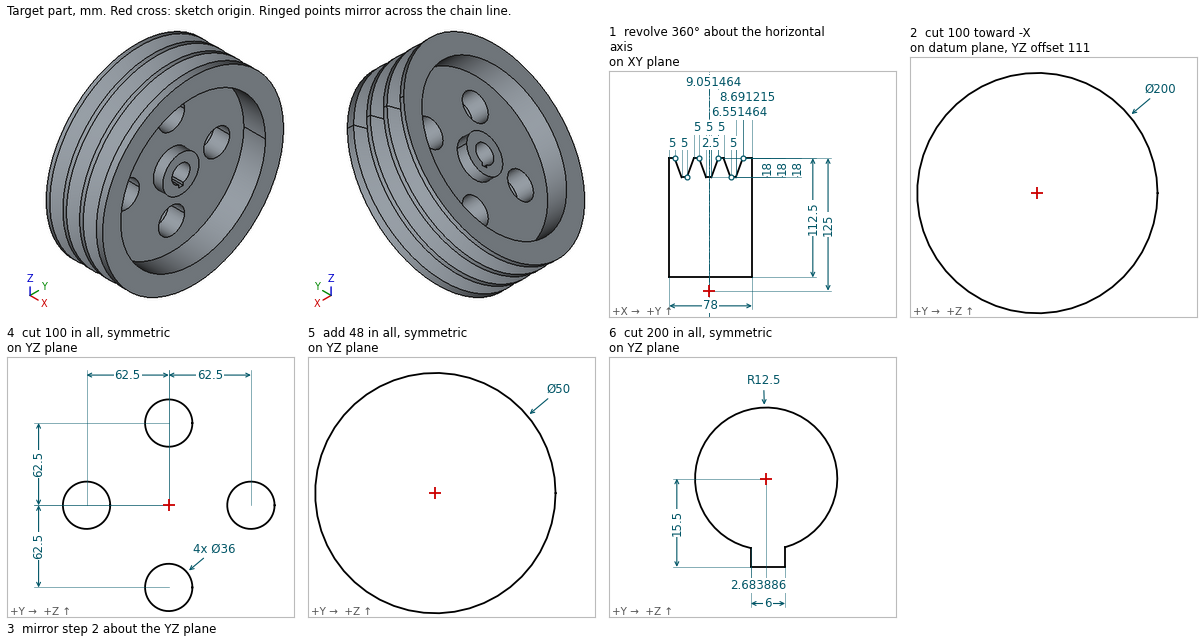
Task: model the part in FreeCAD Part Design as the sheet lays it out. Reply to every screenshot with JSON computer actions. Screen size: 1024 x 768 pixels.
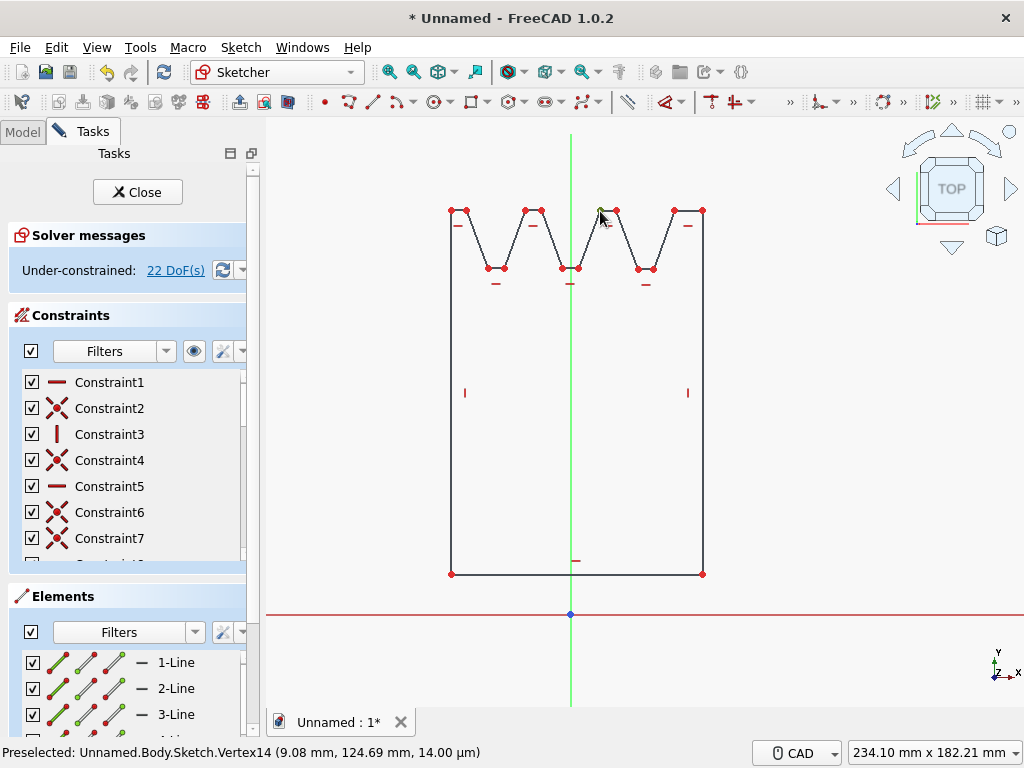
{"action": "left_click", "coordinate": [542, 210]}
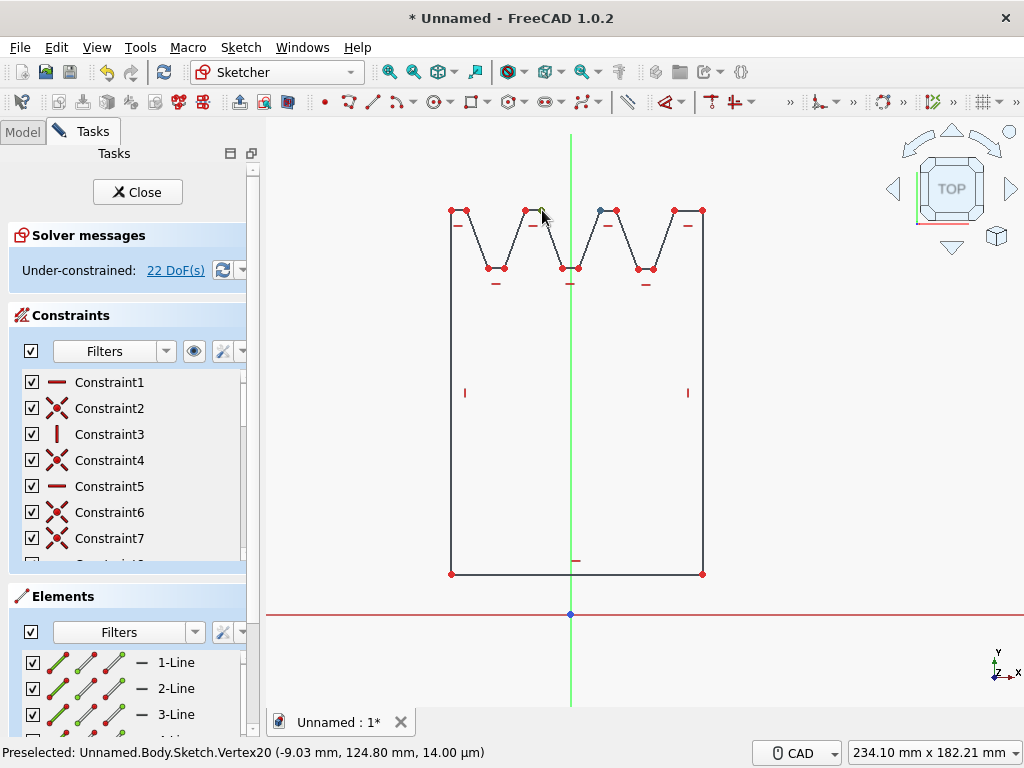
{"action": "left_click", "coordinate": [571, 526]}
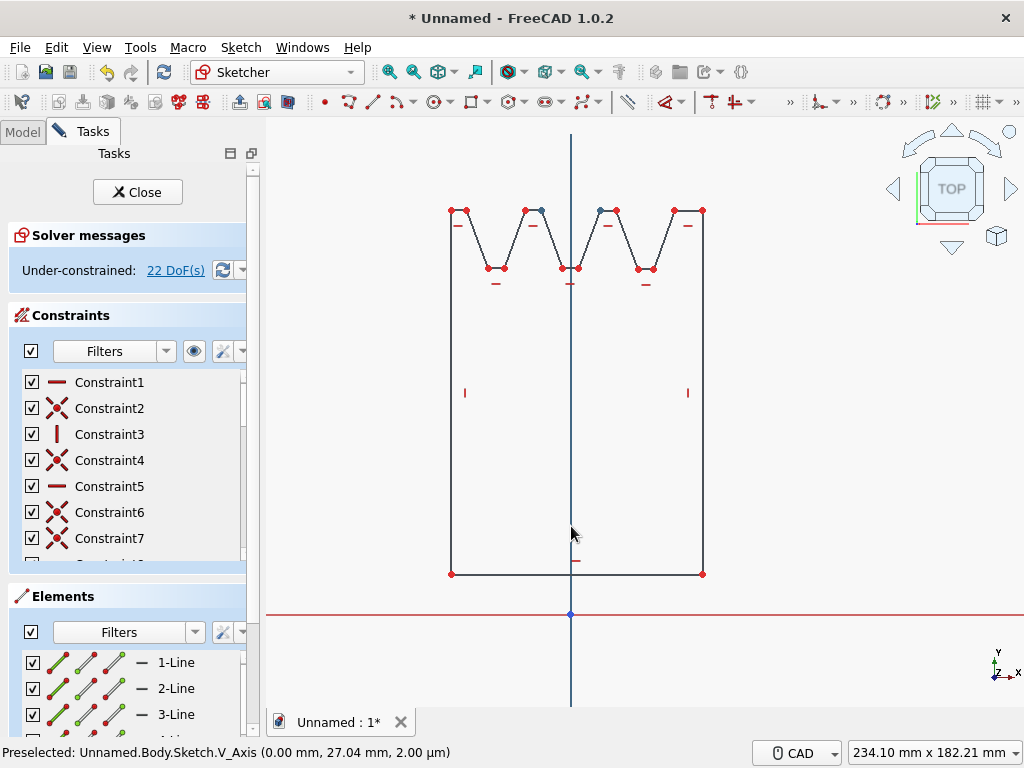
{"action": "key", "text": "s"}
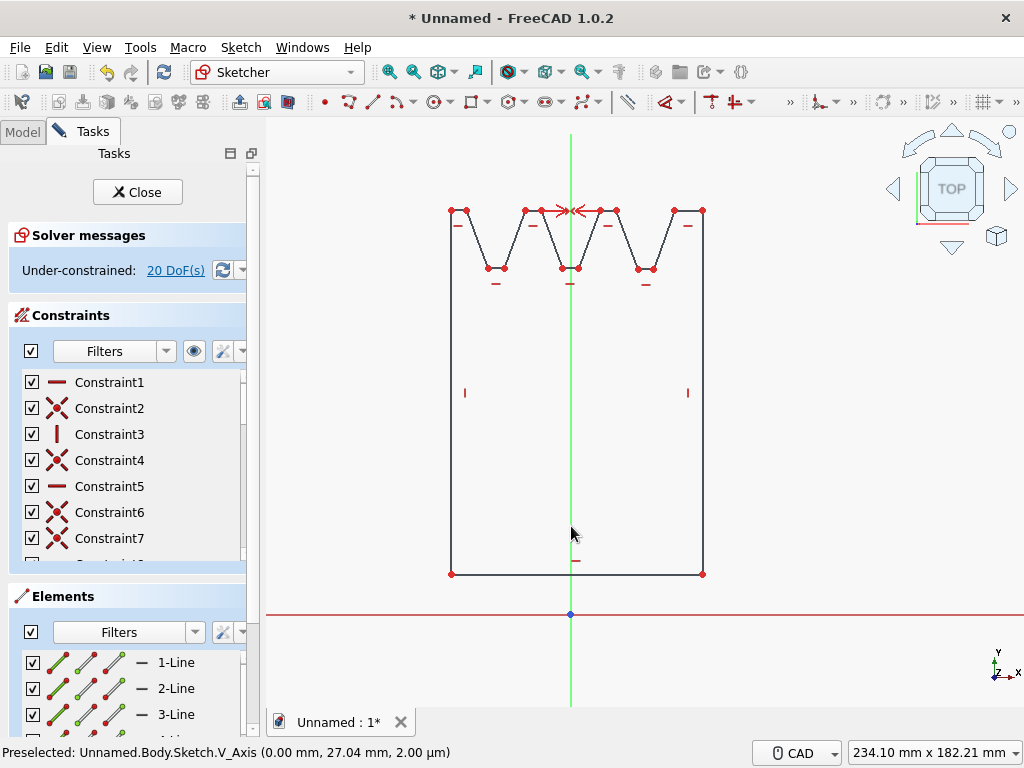
{"action": "left_click", "coordinate": [638, 269]}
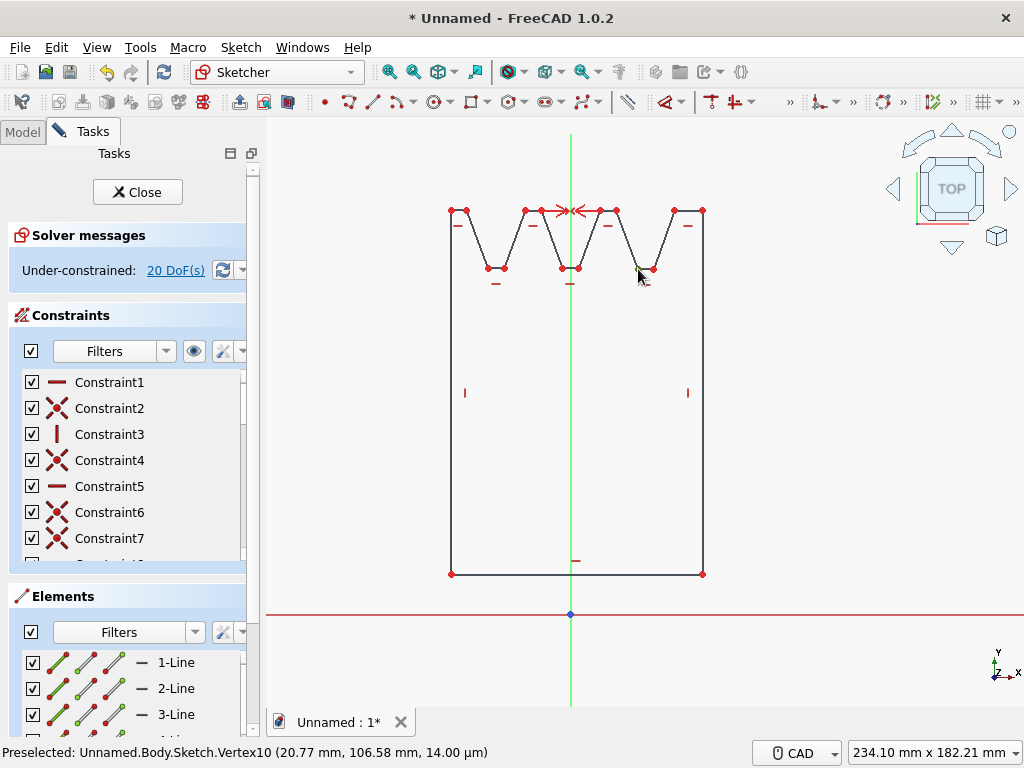
{"action": "left_click", "coordinate": [504, 268]}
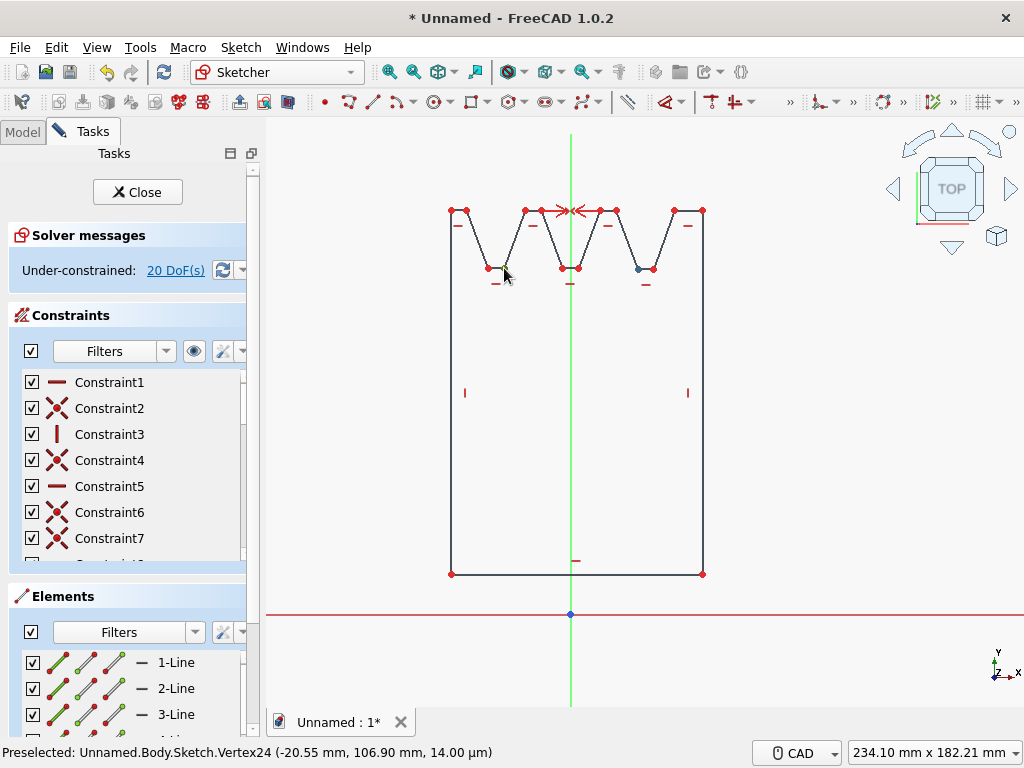
{"action": "left_click", "coordinate": [571, 526]}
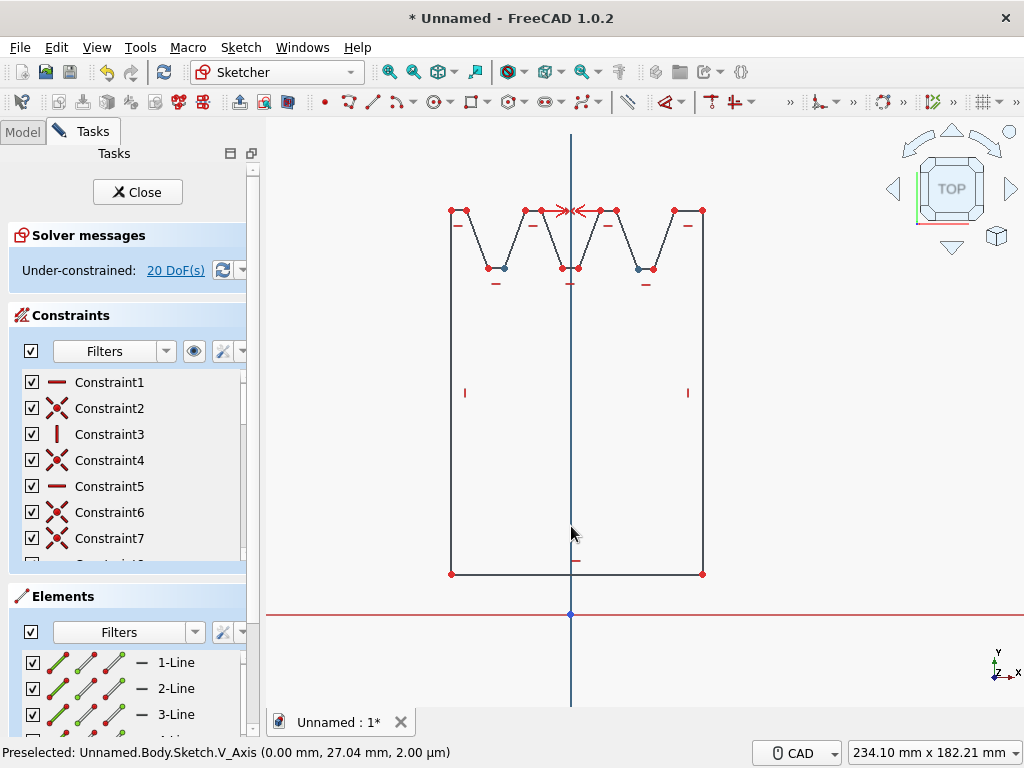
{"action": "key", "text": "s"}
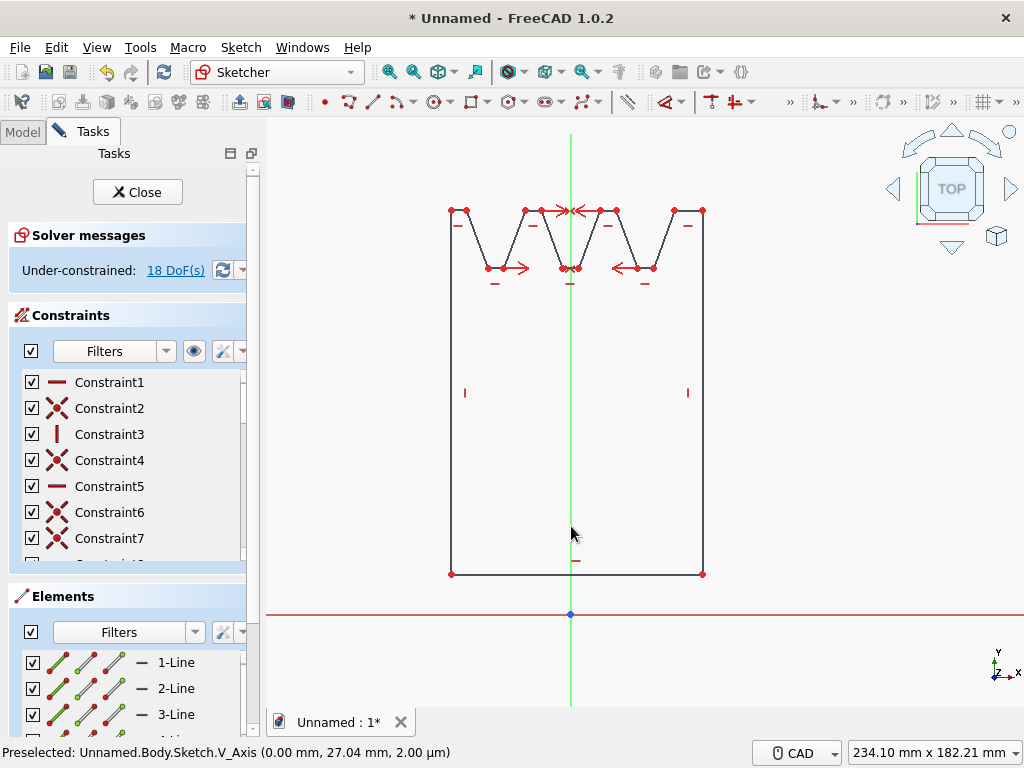
{"action": "left_click", "coordinate": [675, 211]}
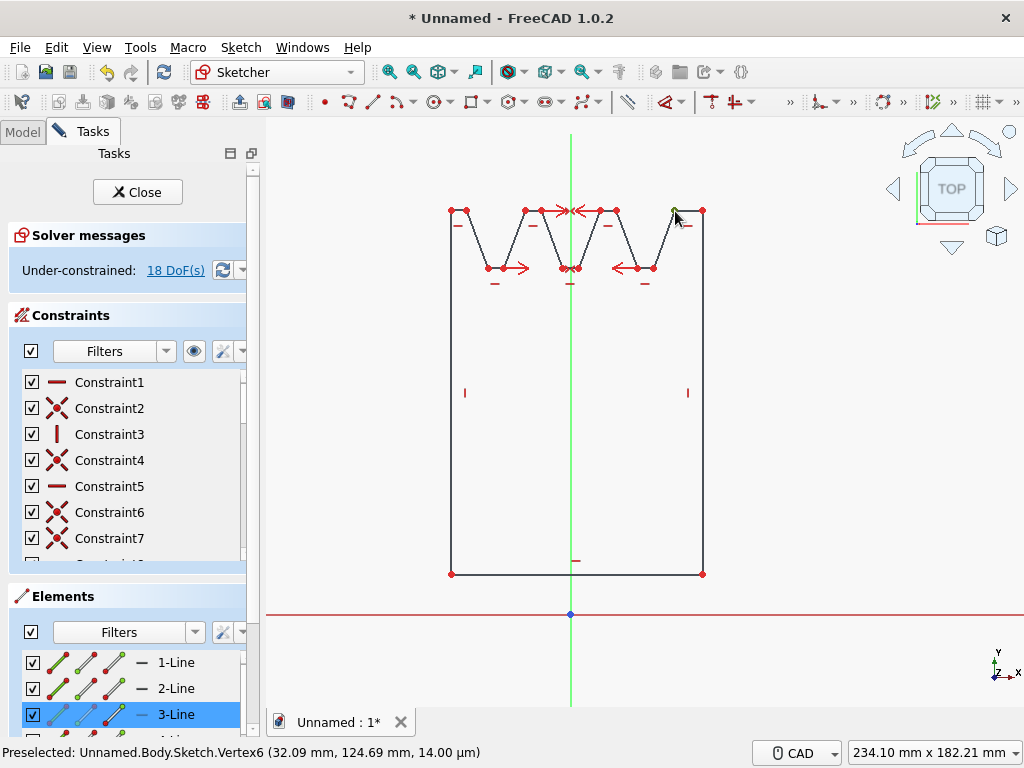
{"action": "left_click", "coordinate": [467, 210]}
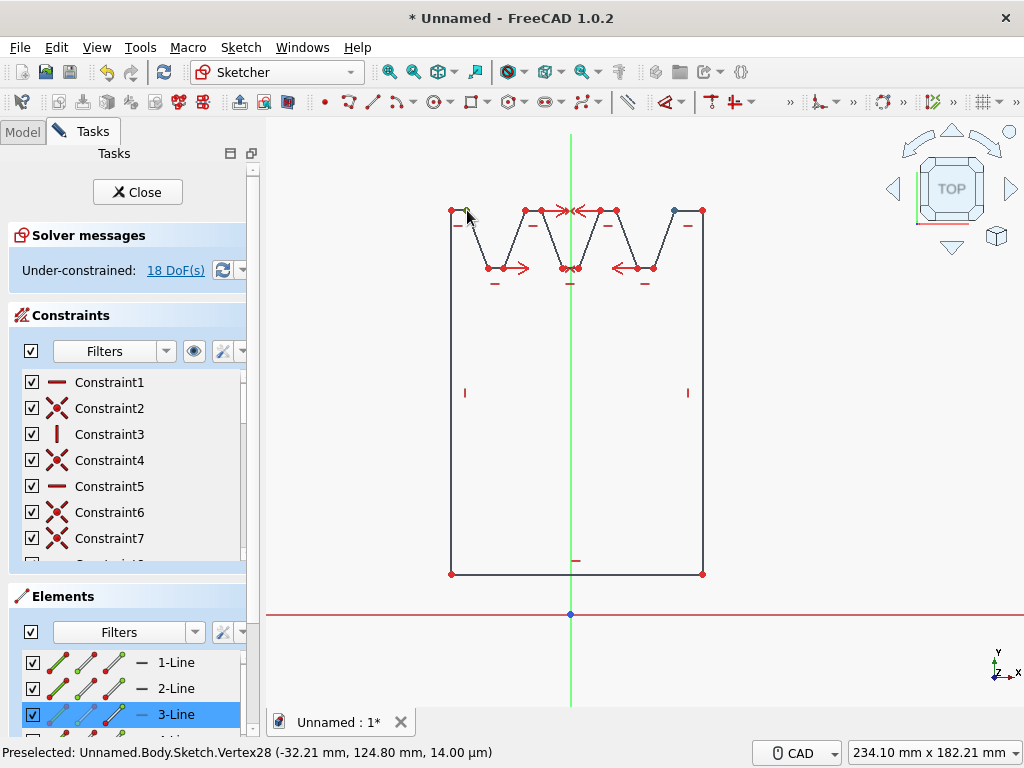
{"action": "left_click", "coordinate": [571, 526]}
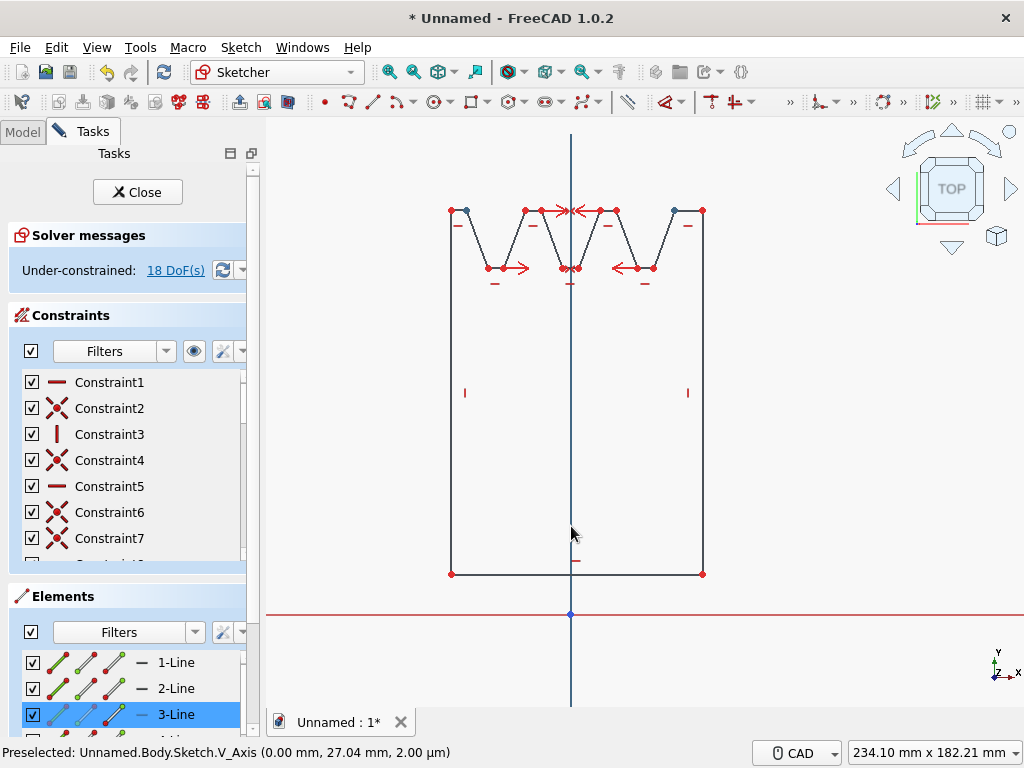
{"action": "key", "text": "s"}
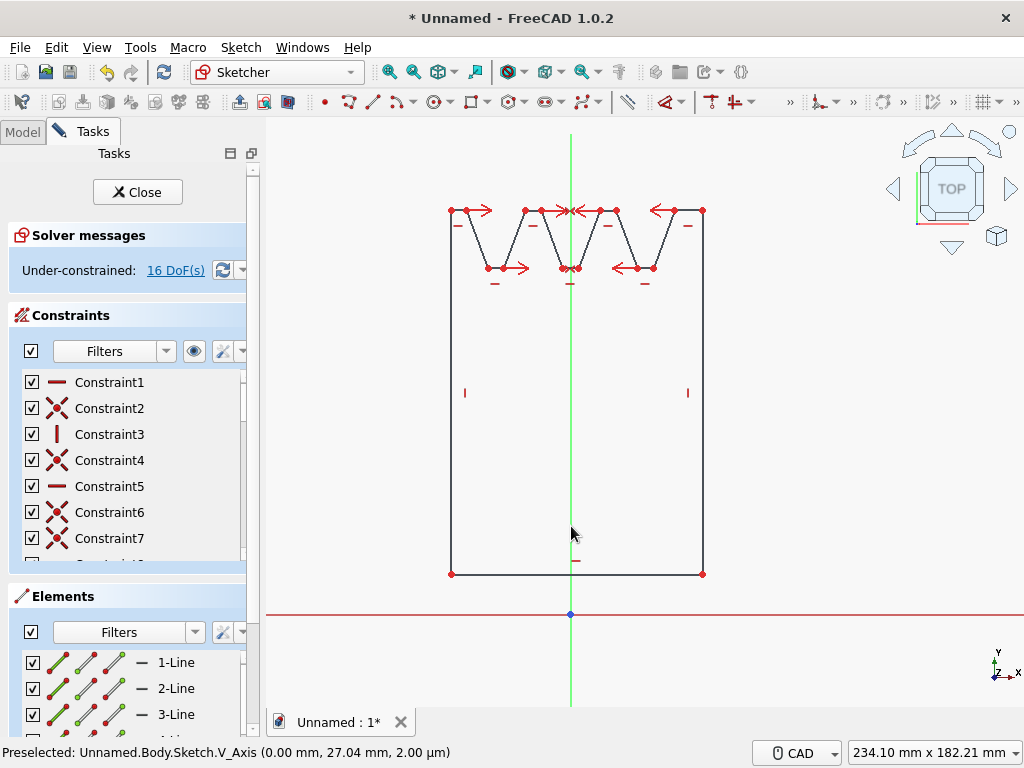
{"action": "scroll", "coordinate": [646, 268], "scroll_direction": "up", "scroll_amount": 5}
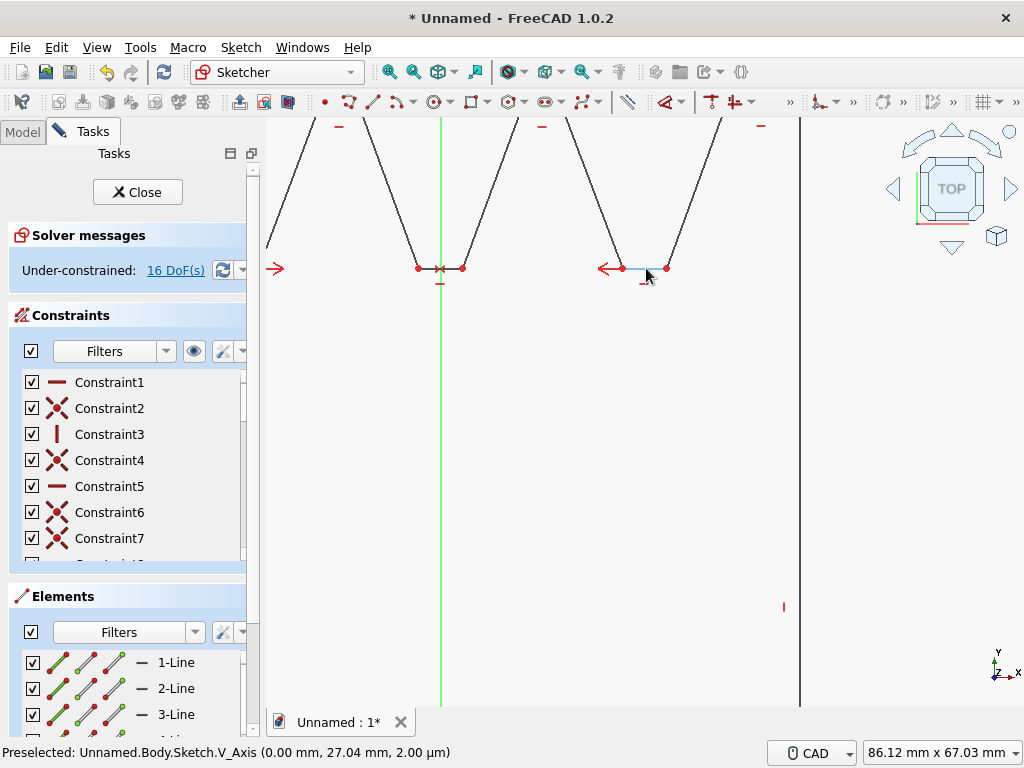
{"action": "left_click", "coordinate": [645, 269]}